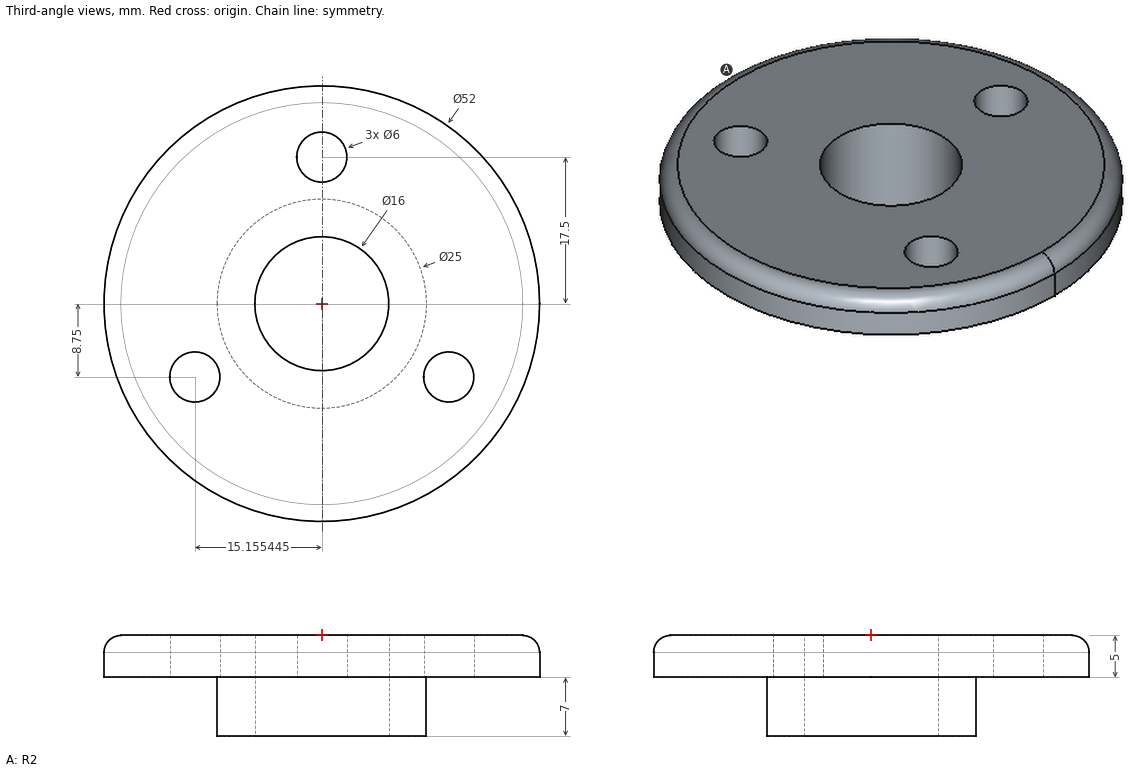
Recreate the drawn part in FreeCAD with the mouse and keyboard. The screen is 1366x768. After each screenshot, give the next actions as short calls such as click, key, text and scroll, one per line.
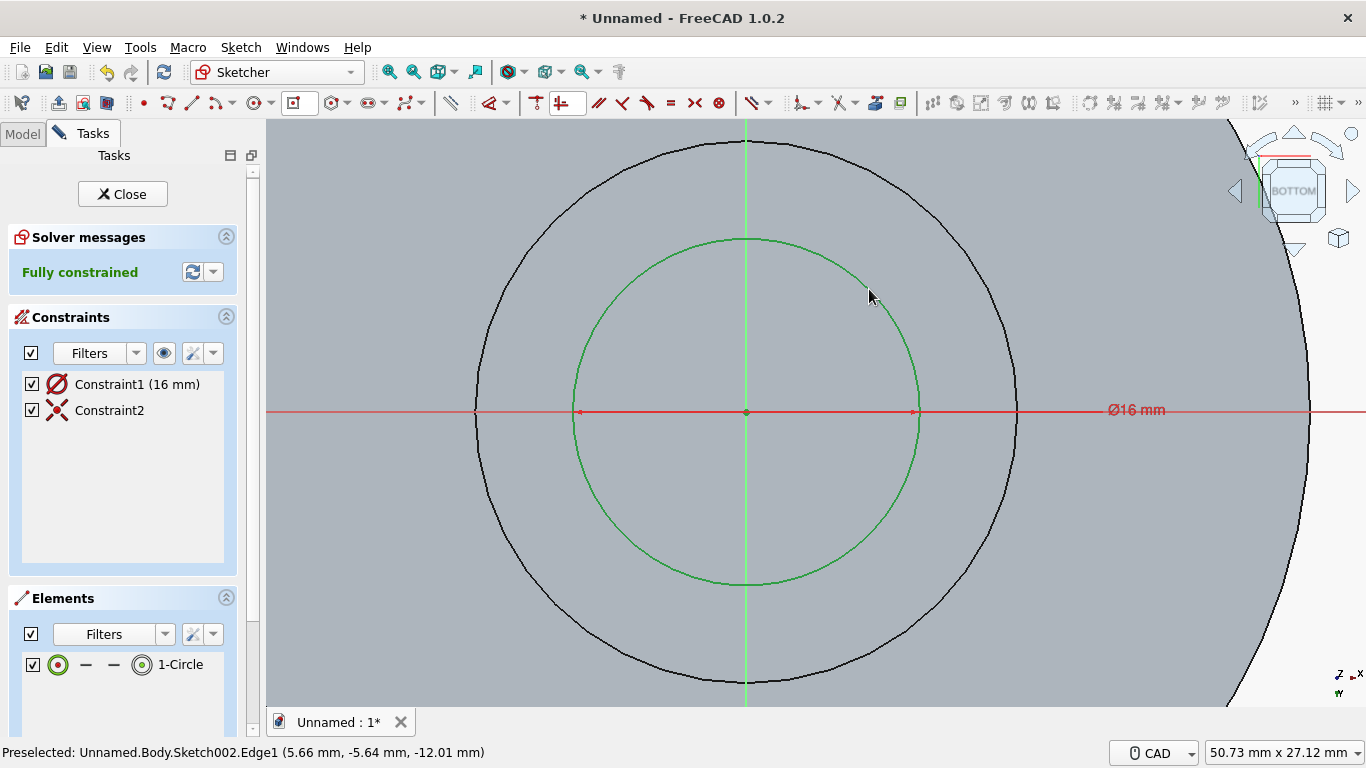
click(123, 194)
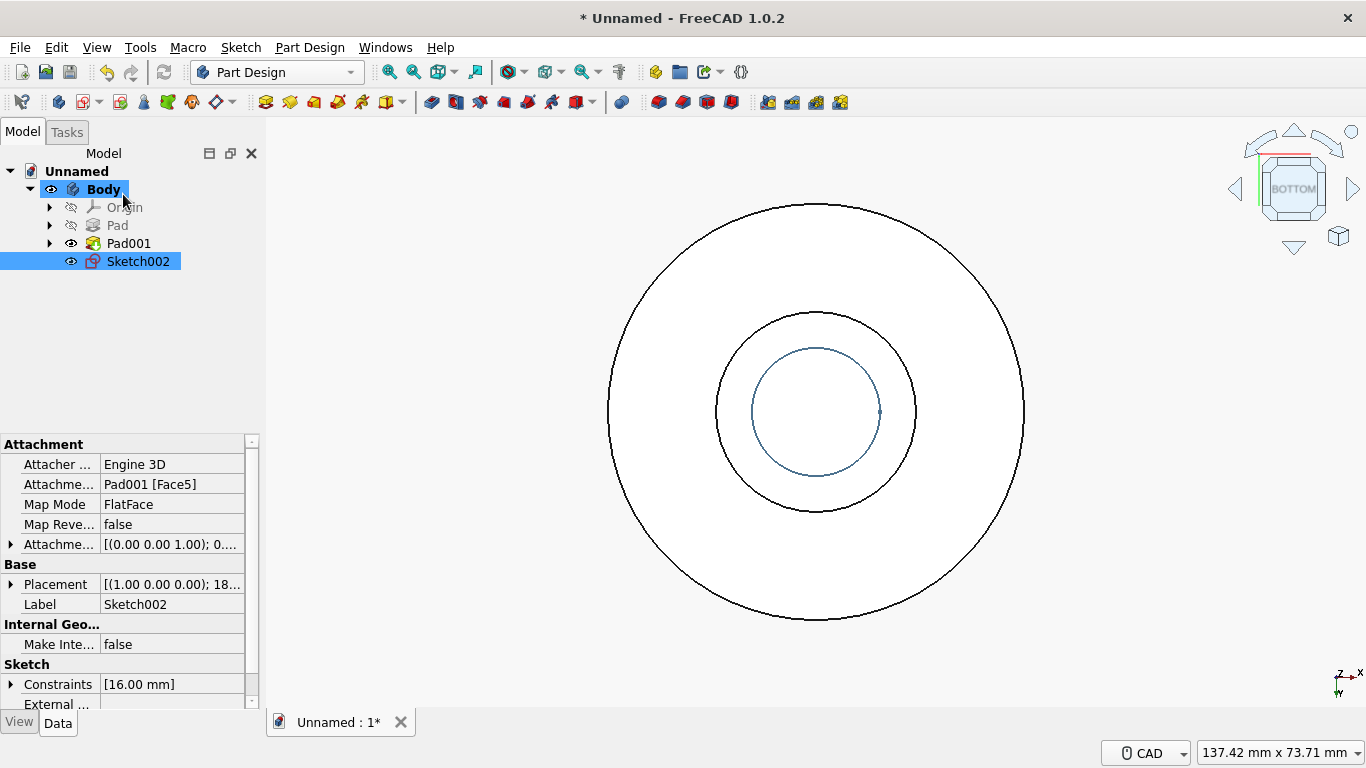
click(432, 102)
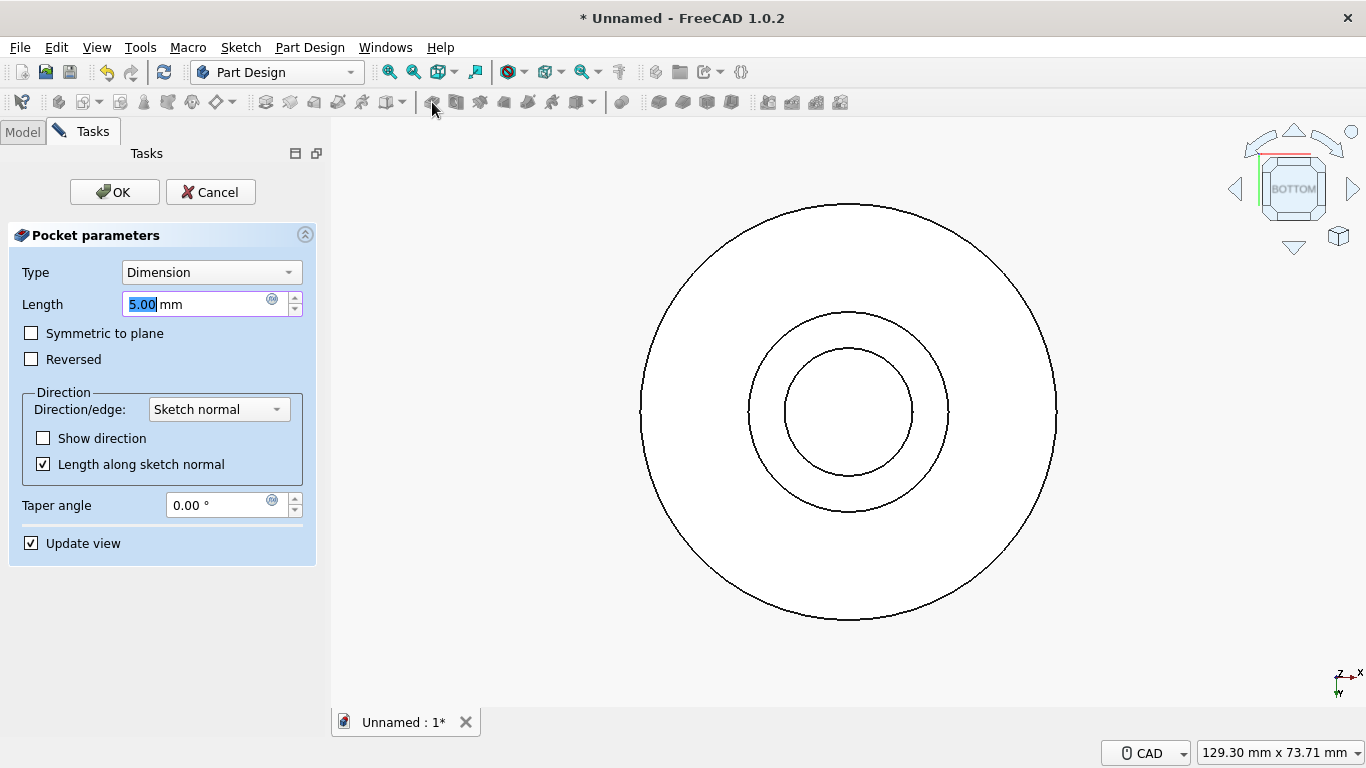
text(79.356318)
key(Tab)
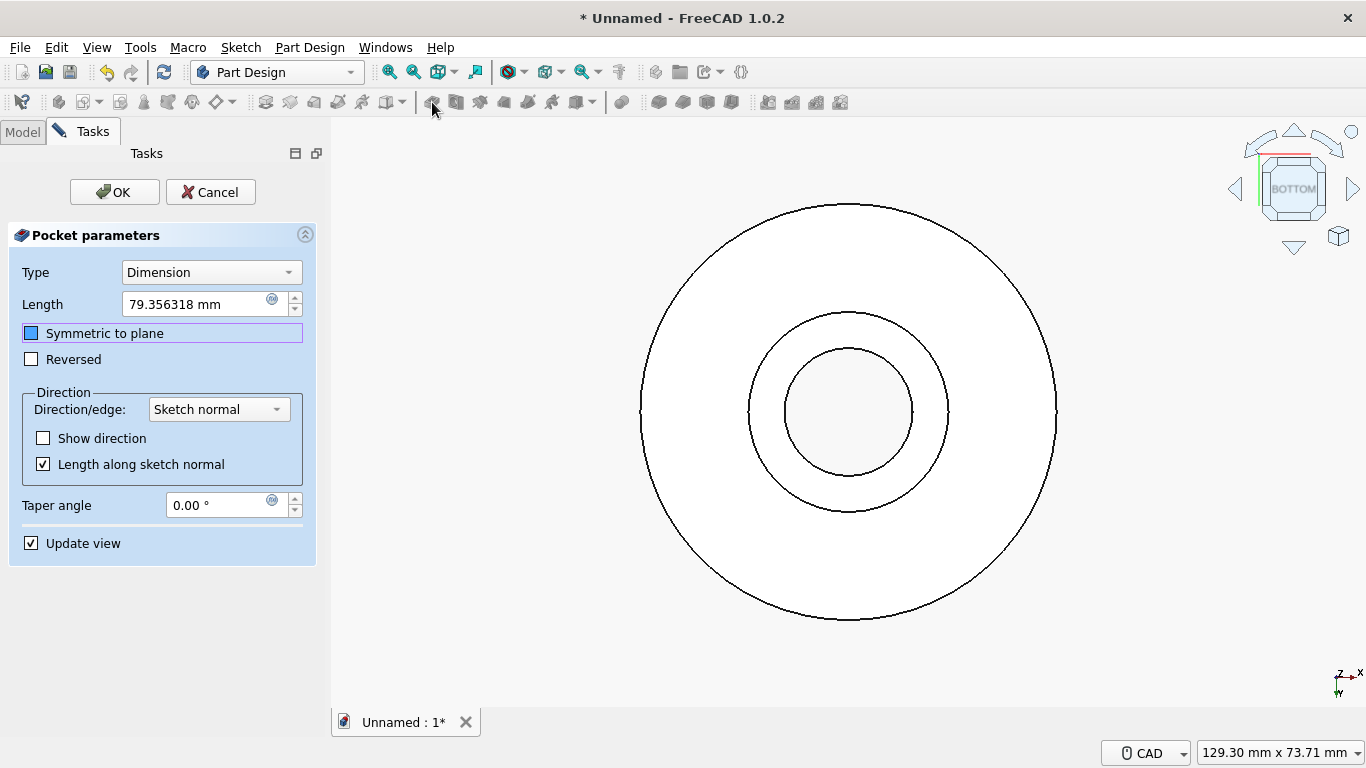
click(30, 333)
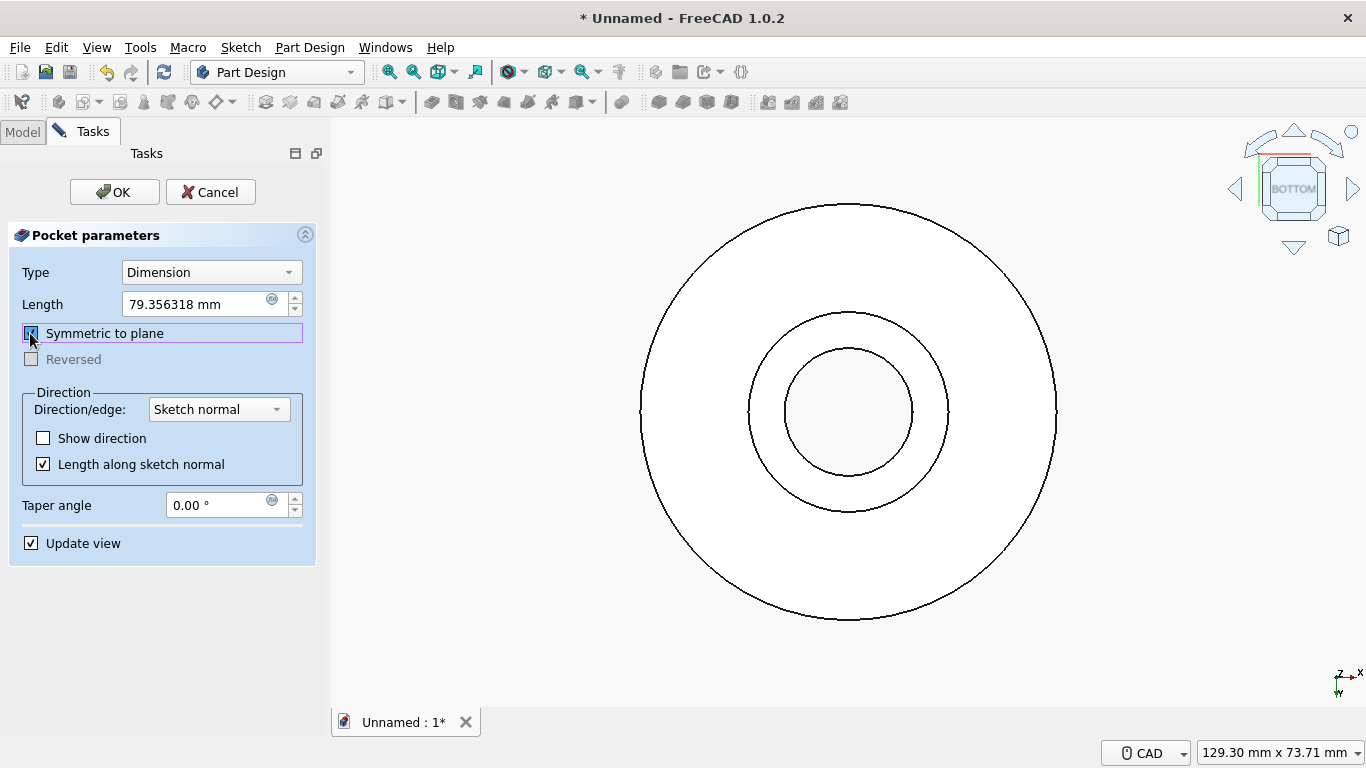
click(115, 192)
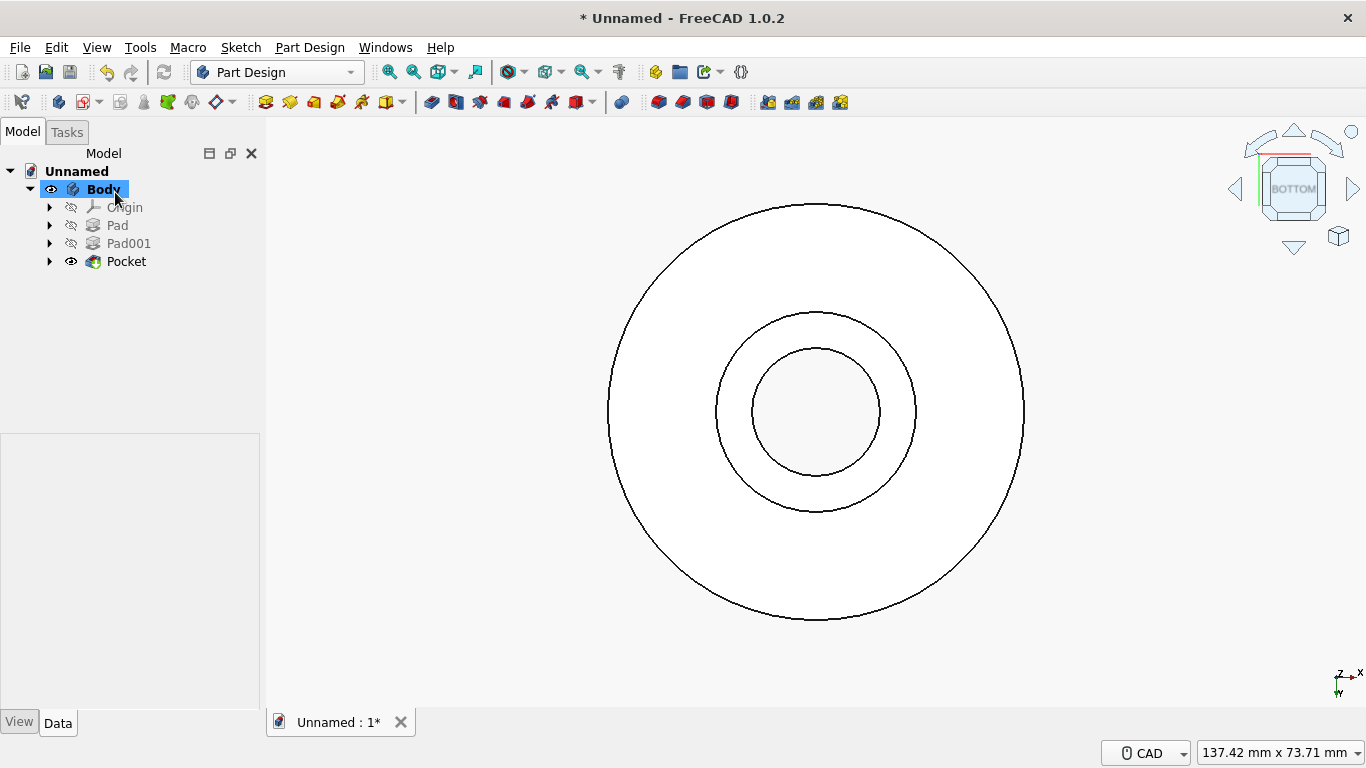
click(935, 530)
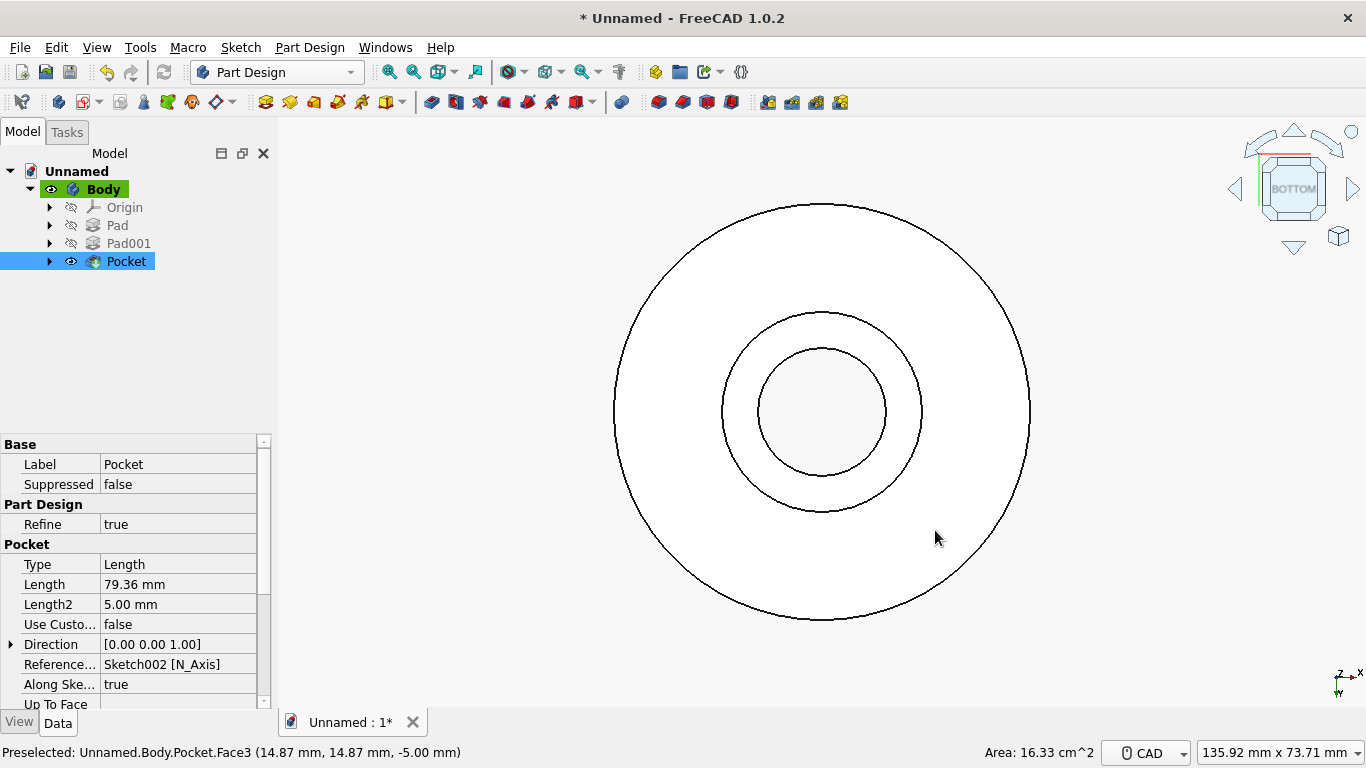
click(84, 102)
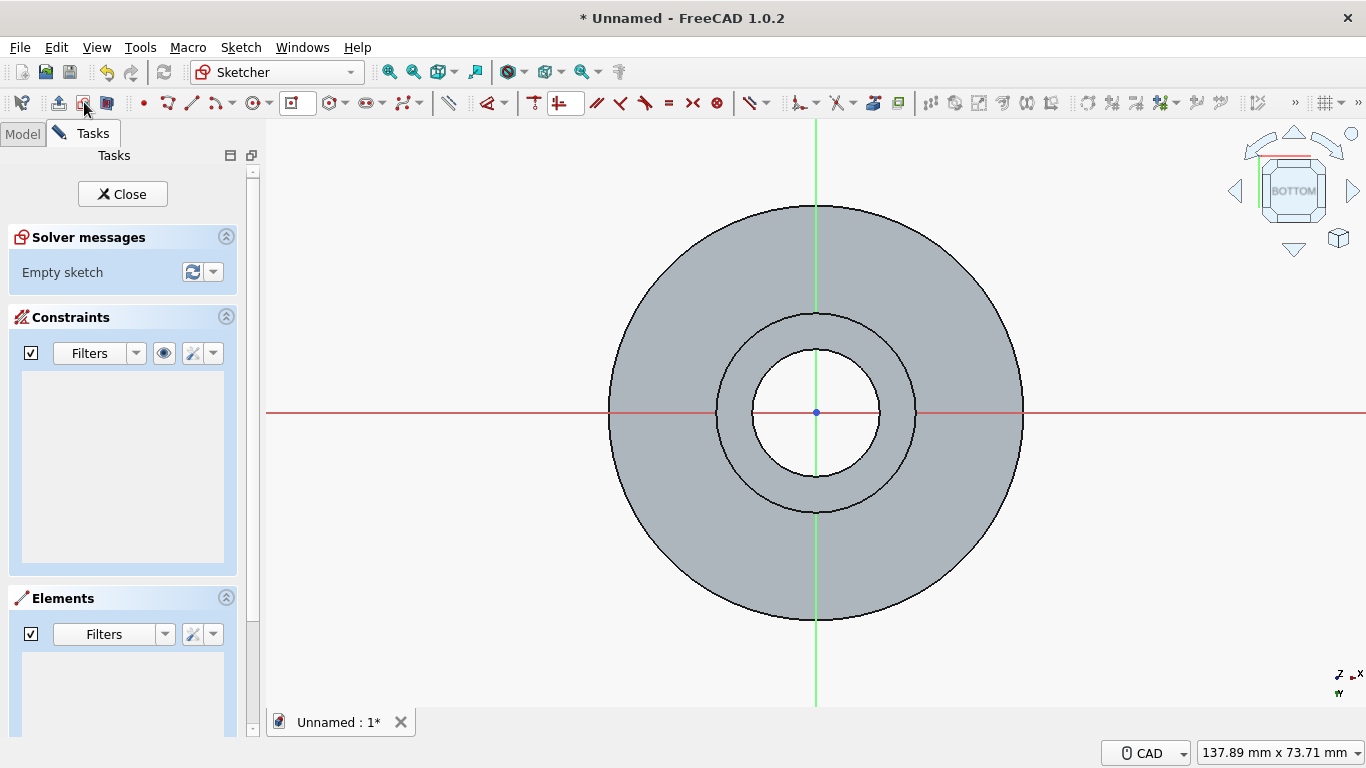
click(108, 104)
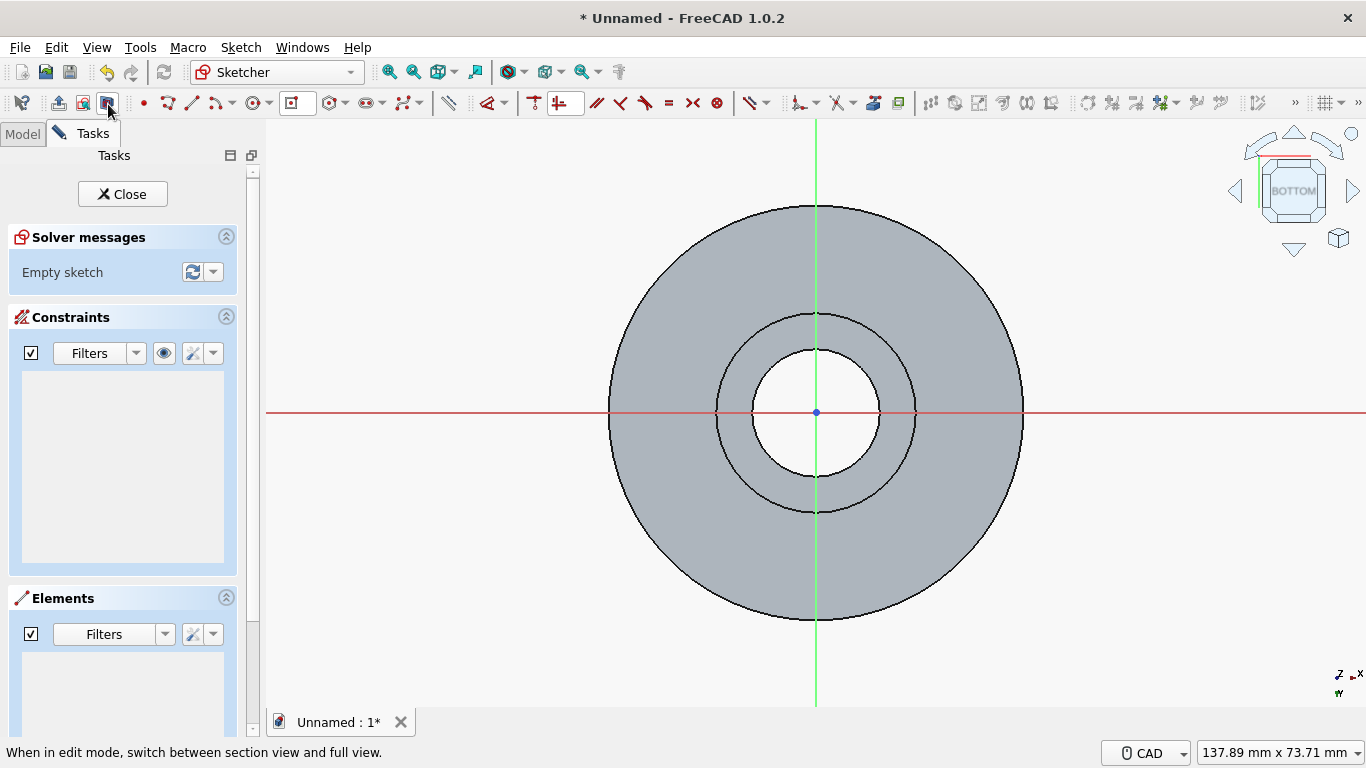
scroll(955, 519, up, 2)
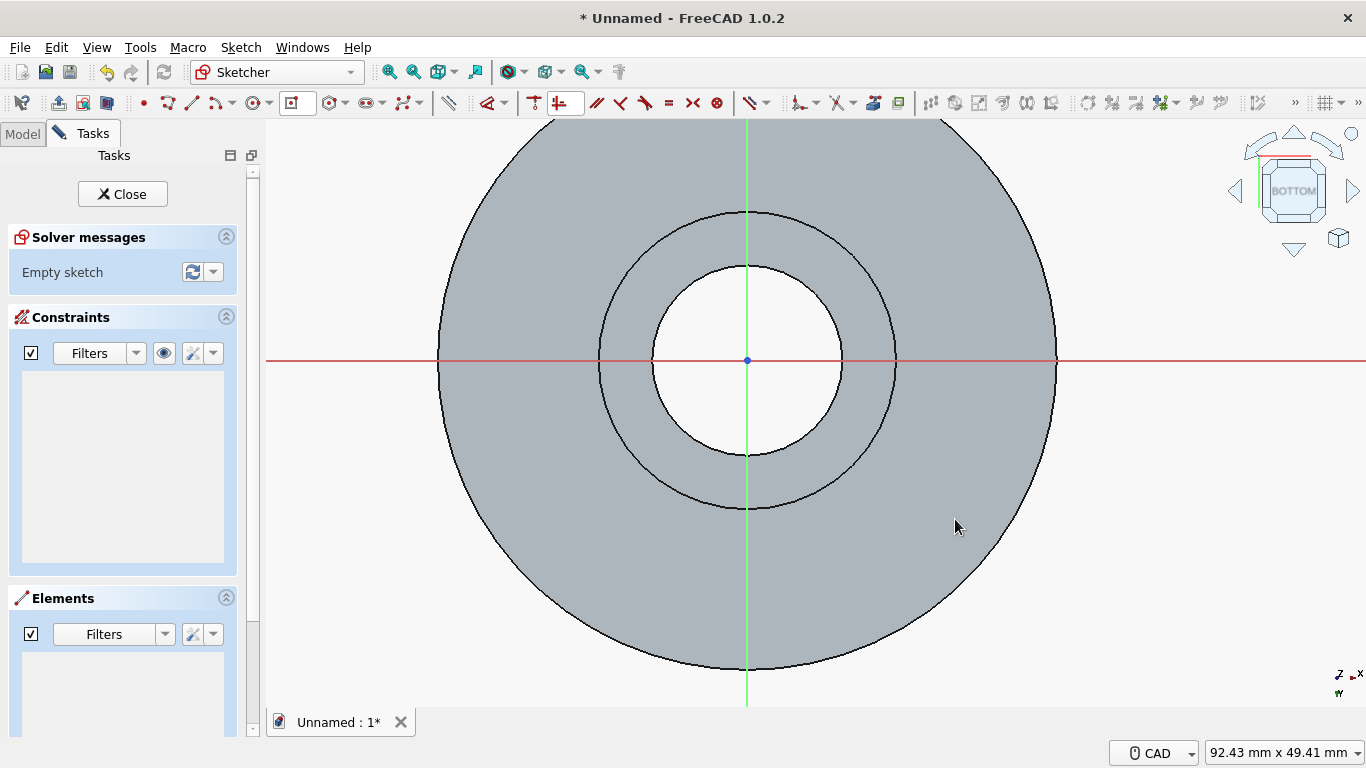
click(254, 104)